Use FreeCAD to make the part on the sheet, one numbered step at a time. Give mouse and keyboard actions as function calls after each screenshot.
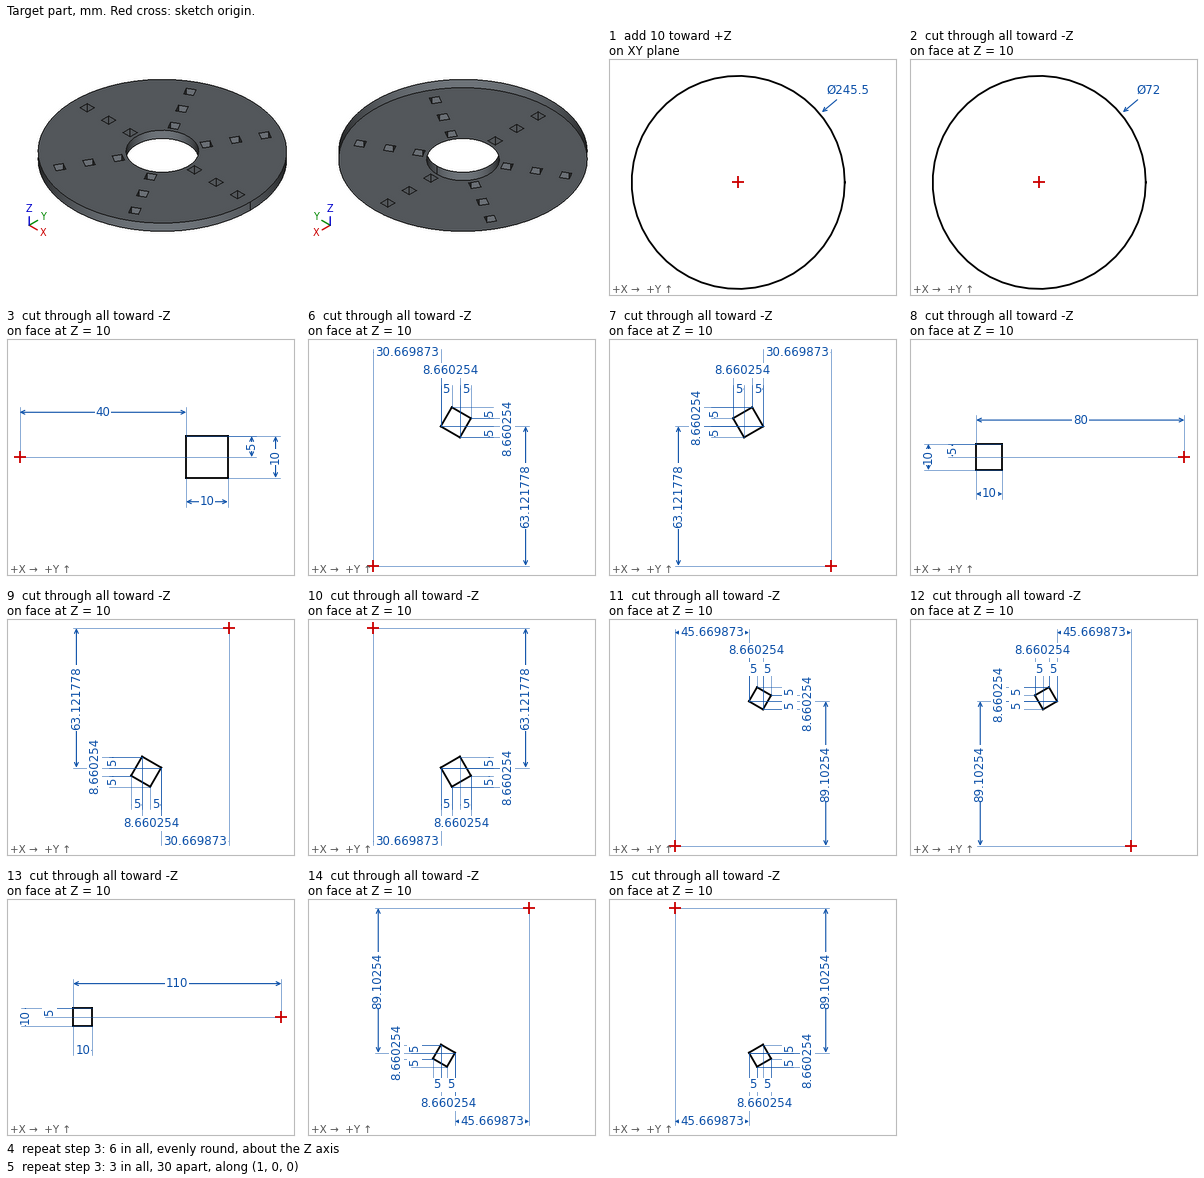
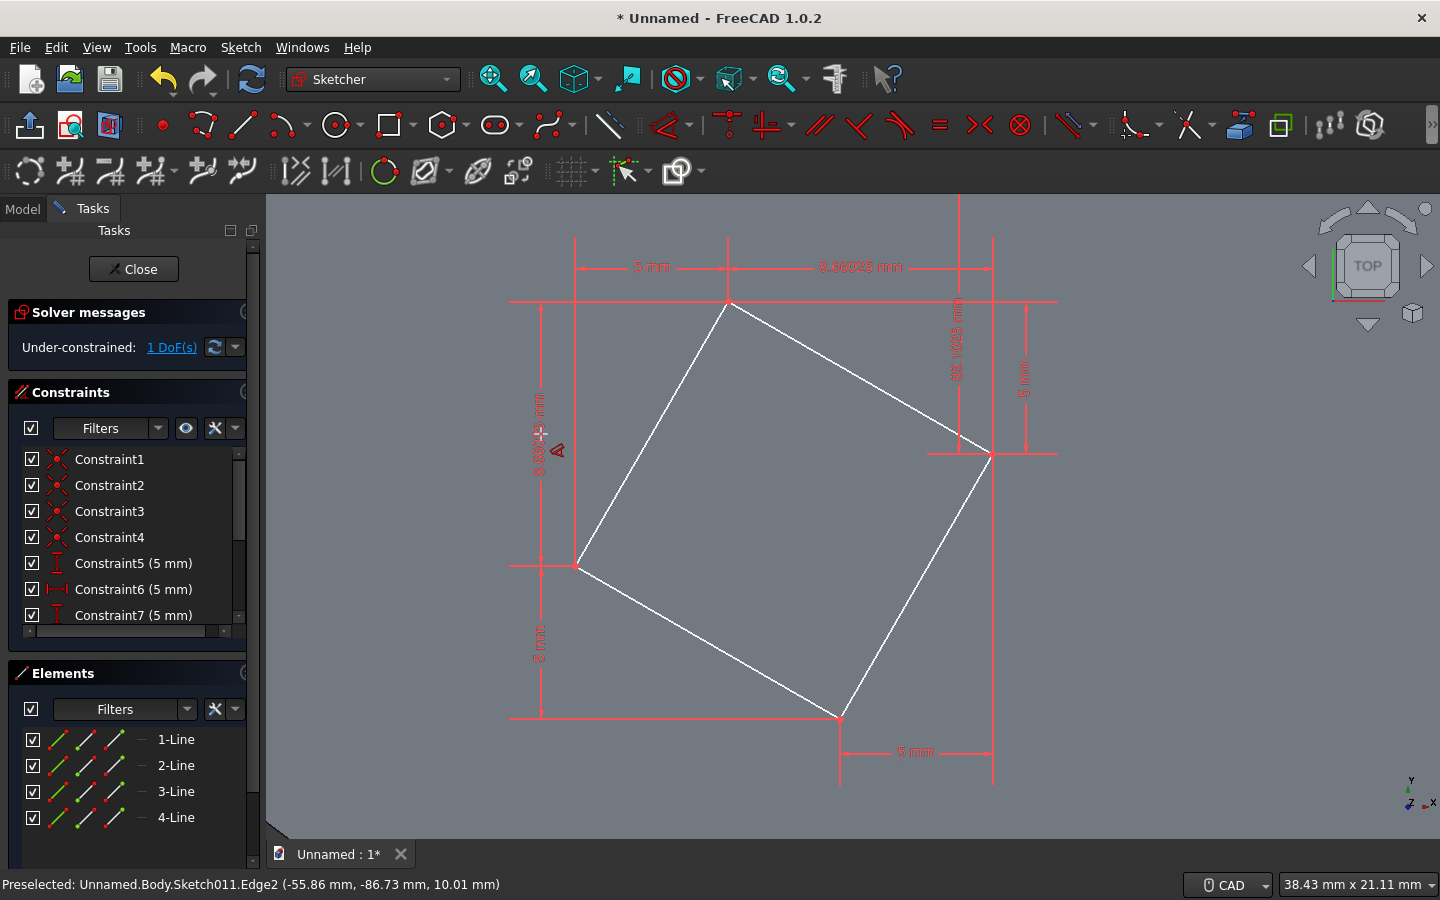
click(993, 454)
click(1134, 488)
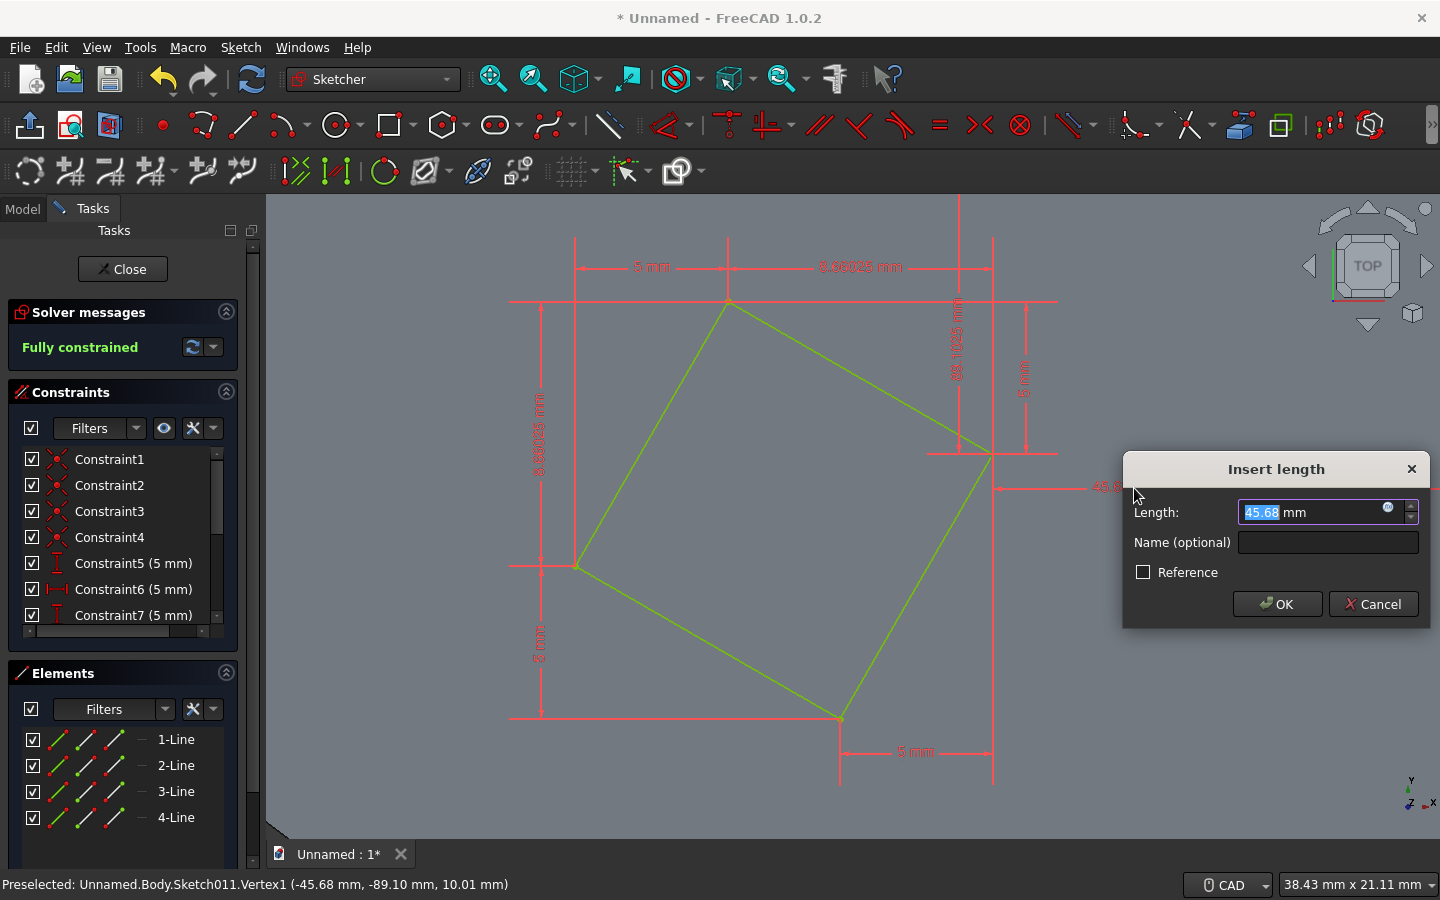
text(45.669873)
key(Return)
key(Escape)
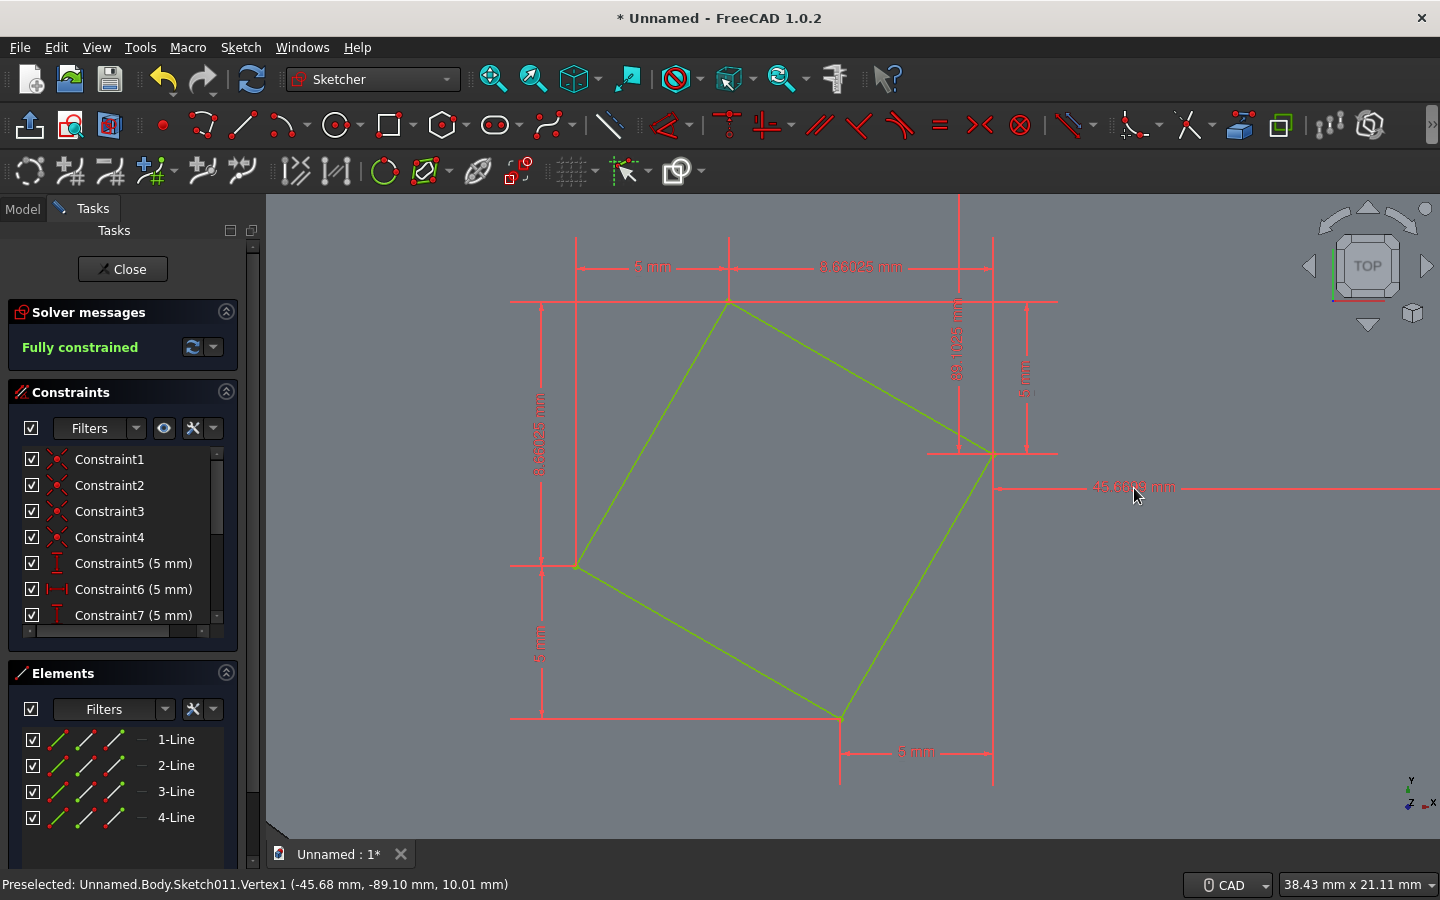
click(123, 269)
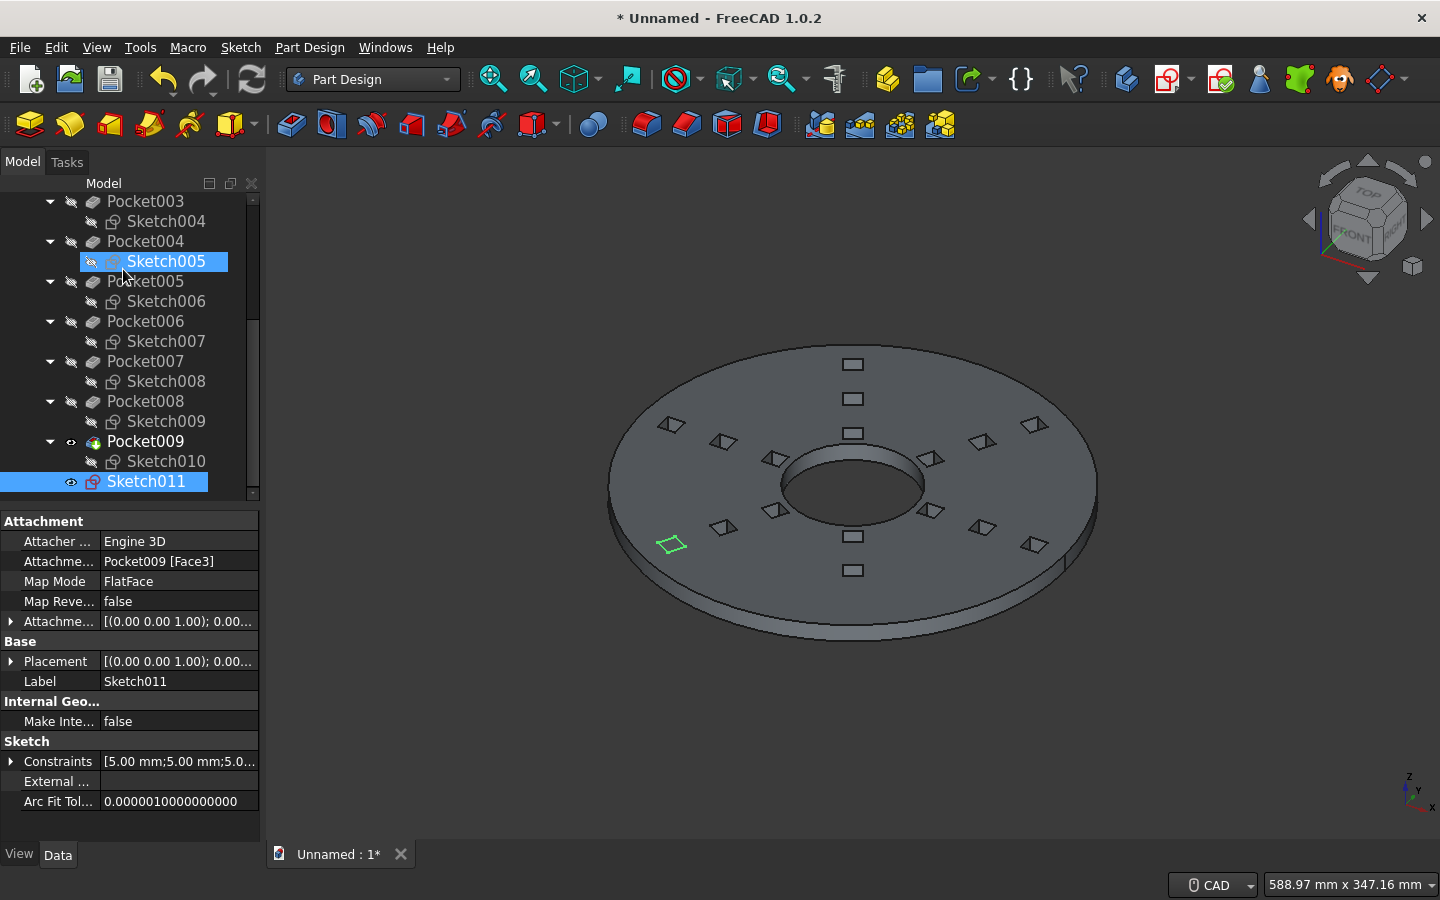
click(292, 124)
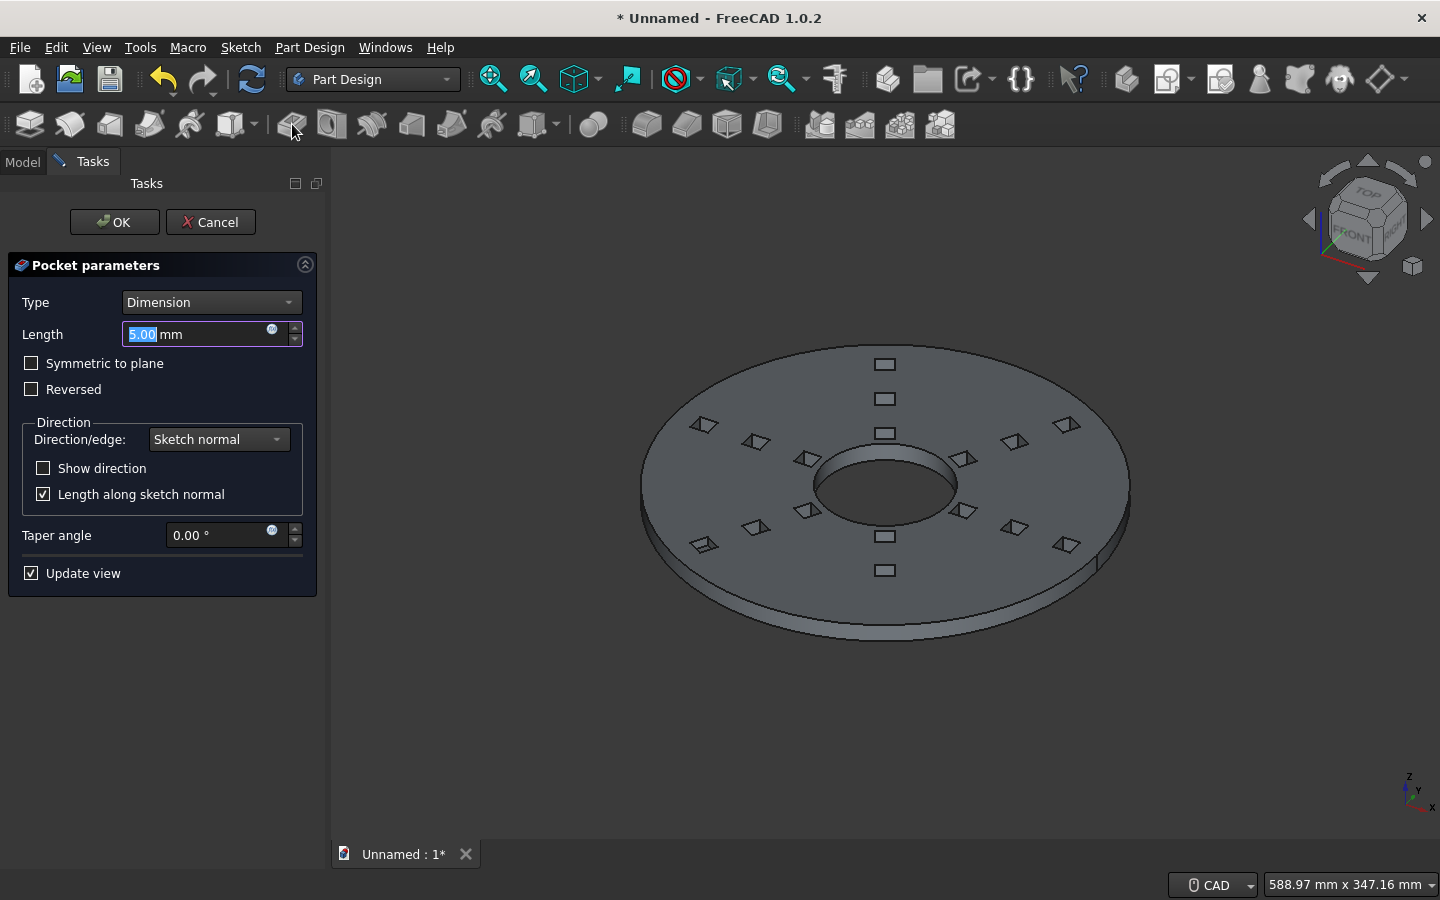
click(212, 302)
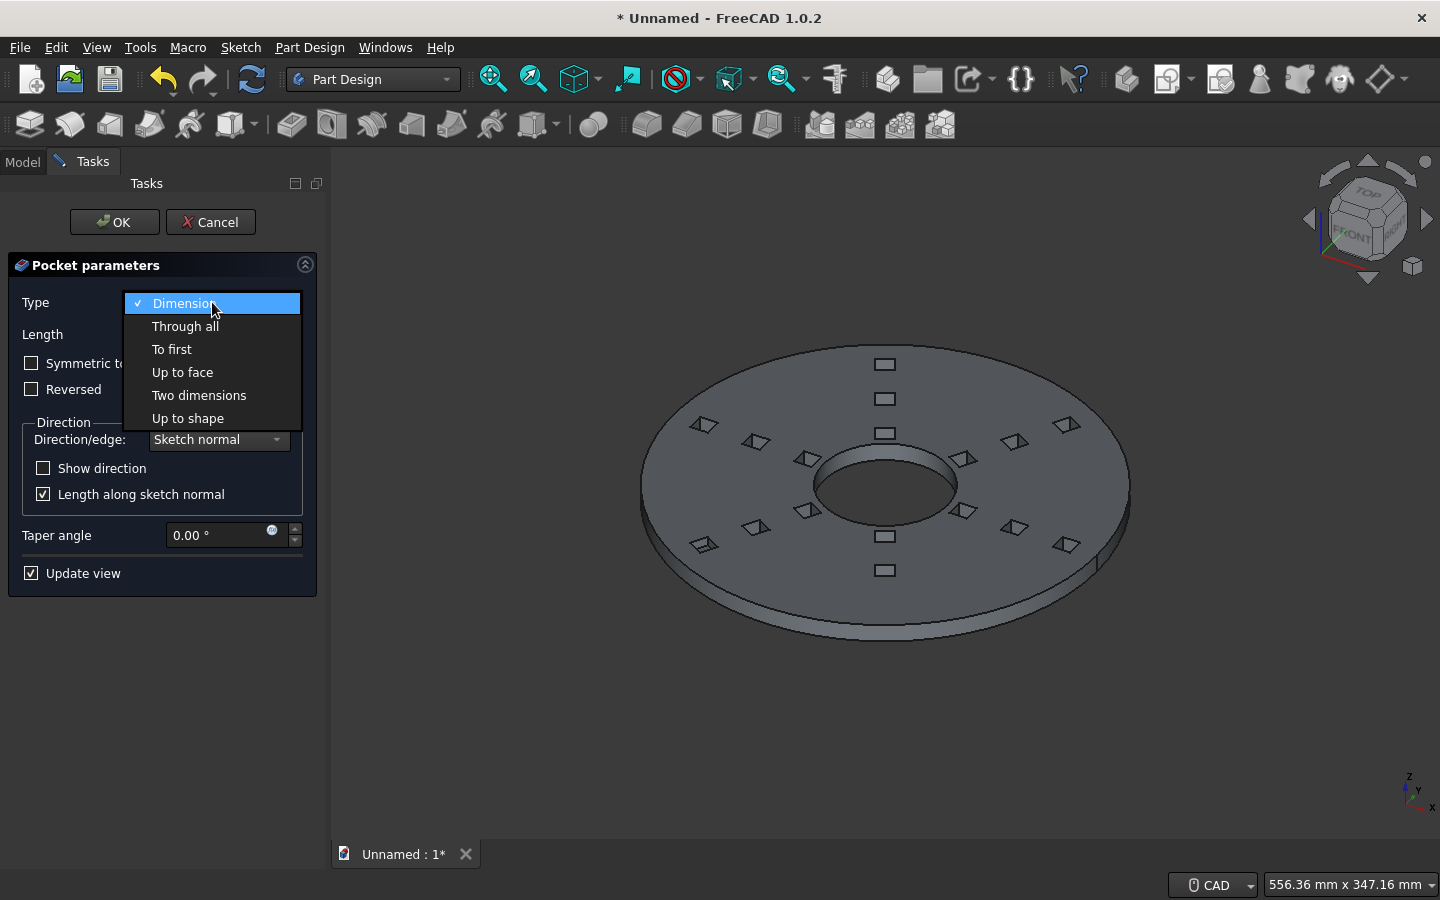
click(212, 326)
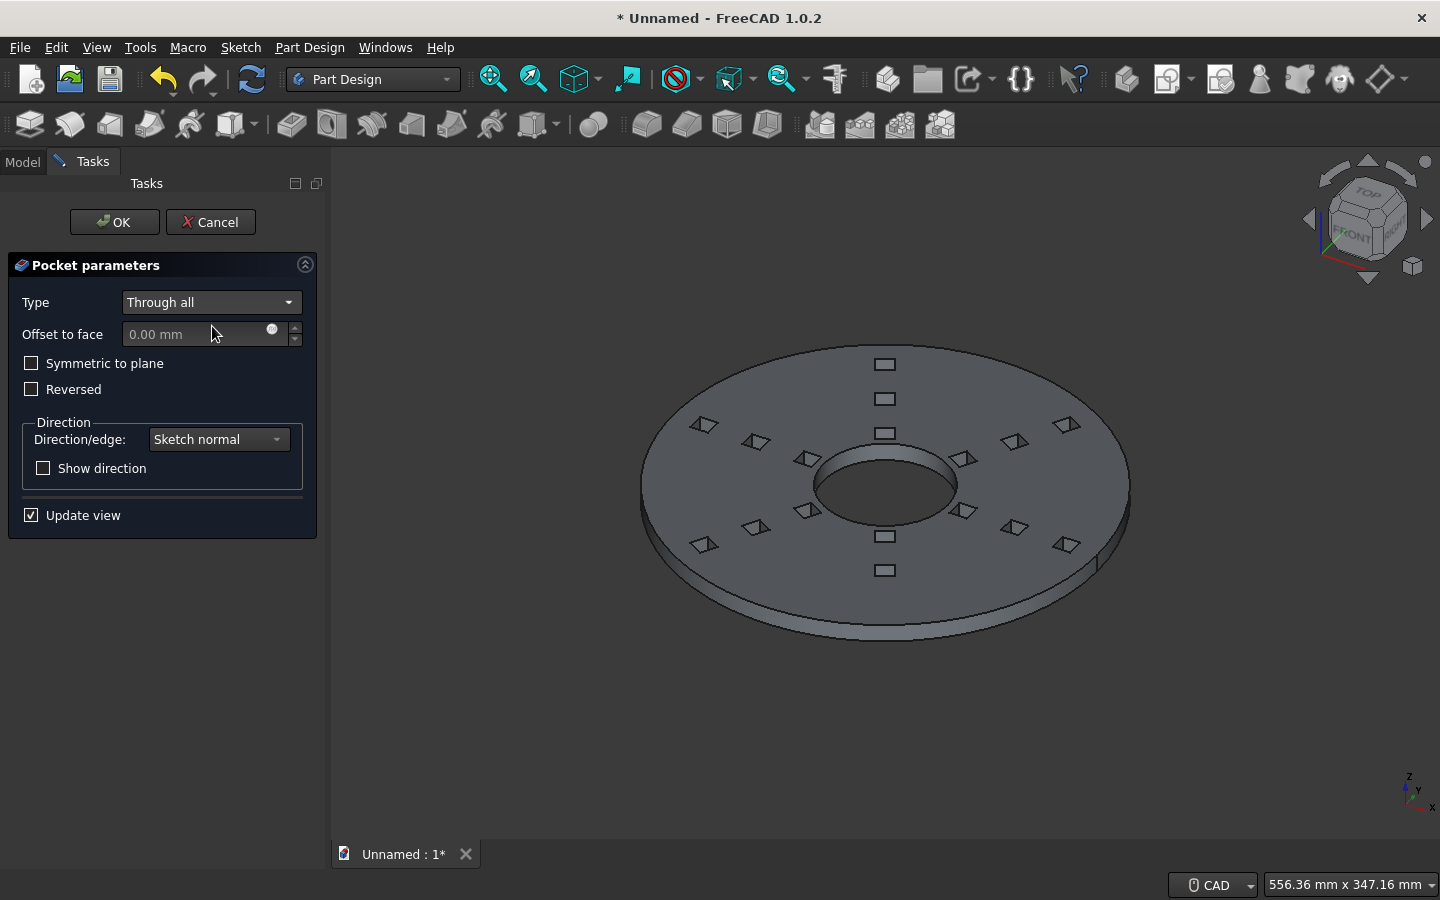
click(115, 222)